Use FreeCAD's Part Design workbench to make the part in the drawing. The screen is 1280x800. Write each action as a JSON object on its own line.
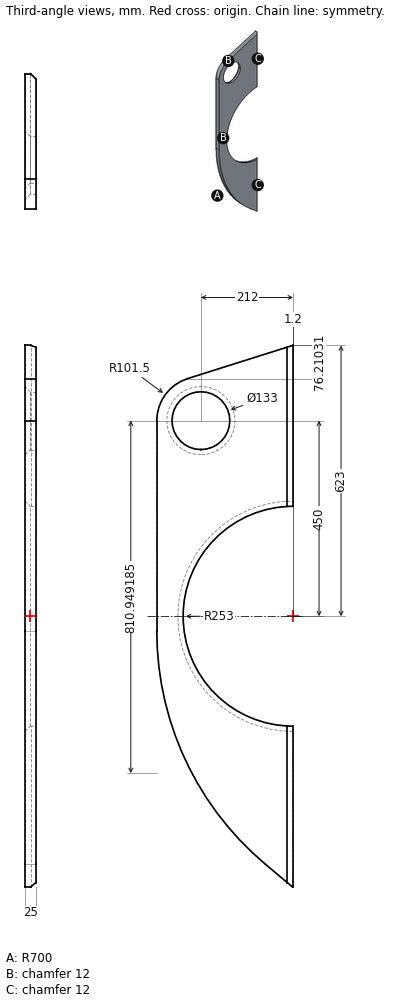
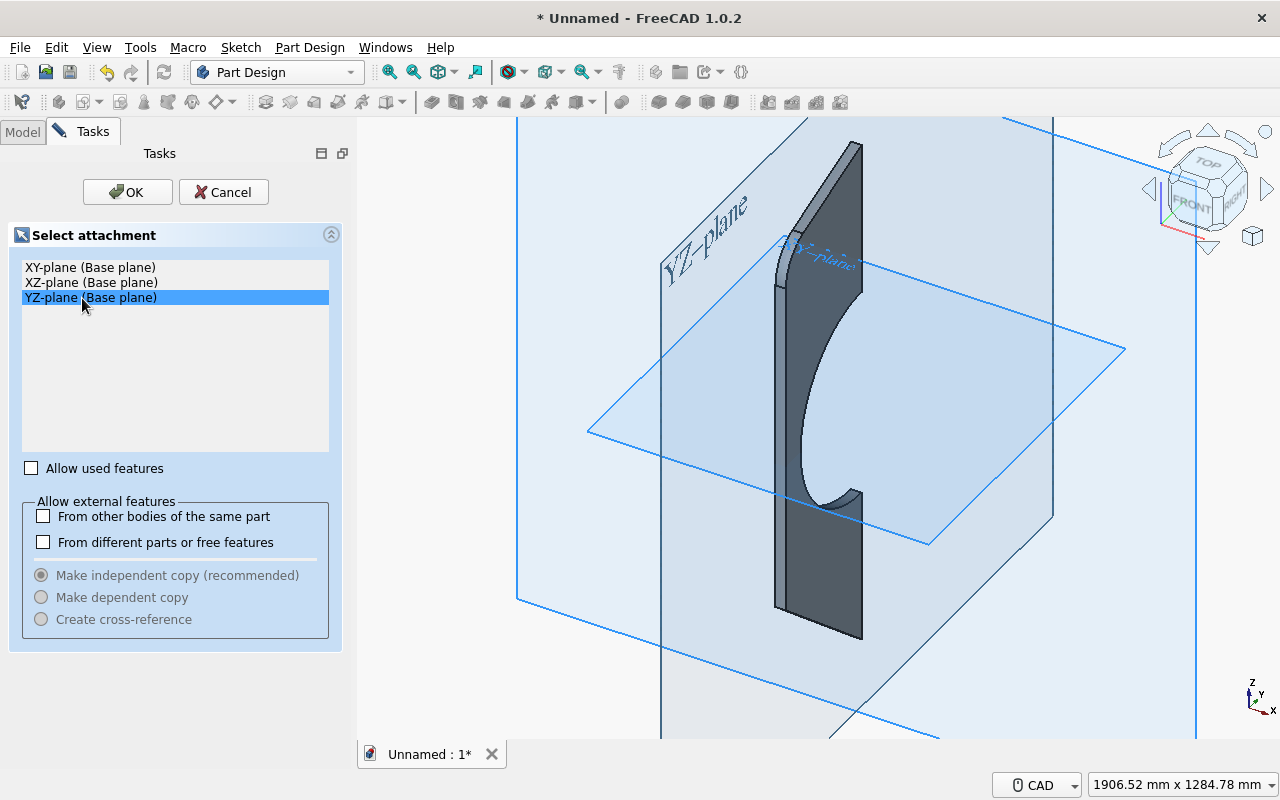
{"action": "left_click", "coordinate": [128, 192]}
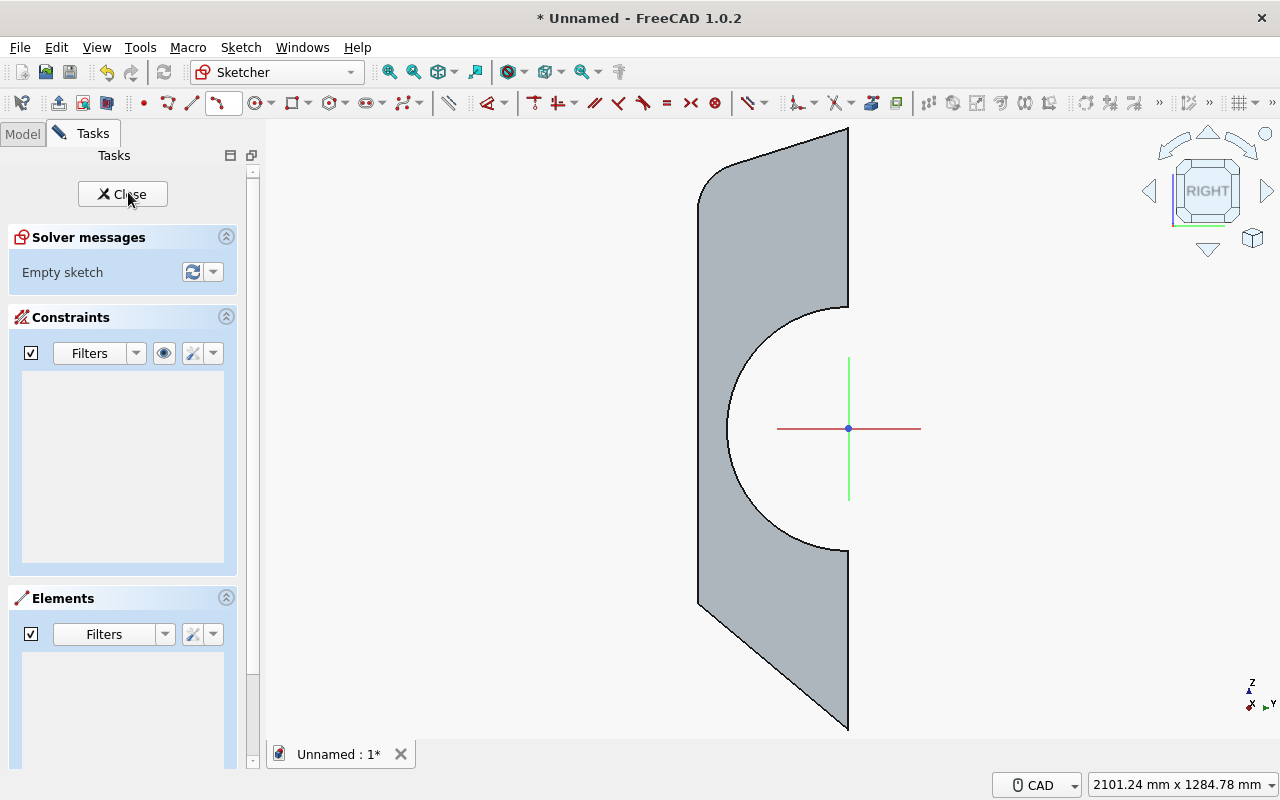
{"action": "left_click", "coordinate": [108, 104]}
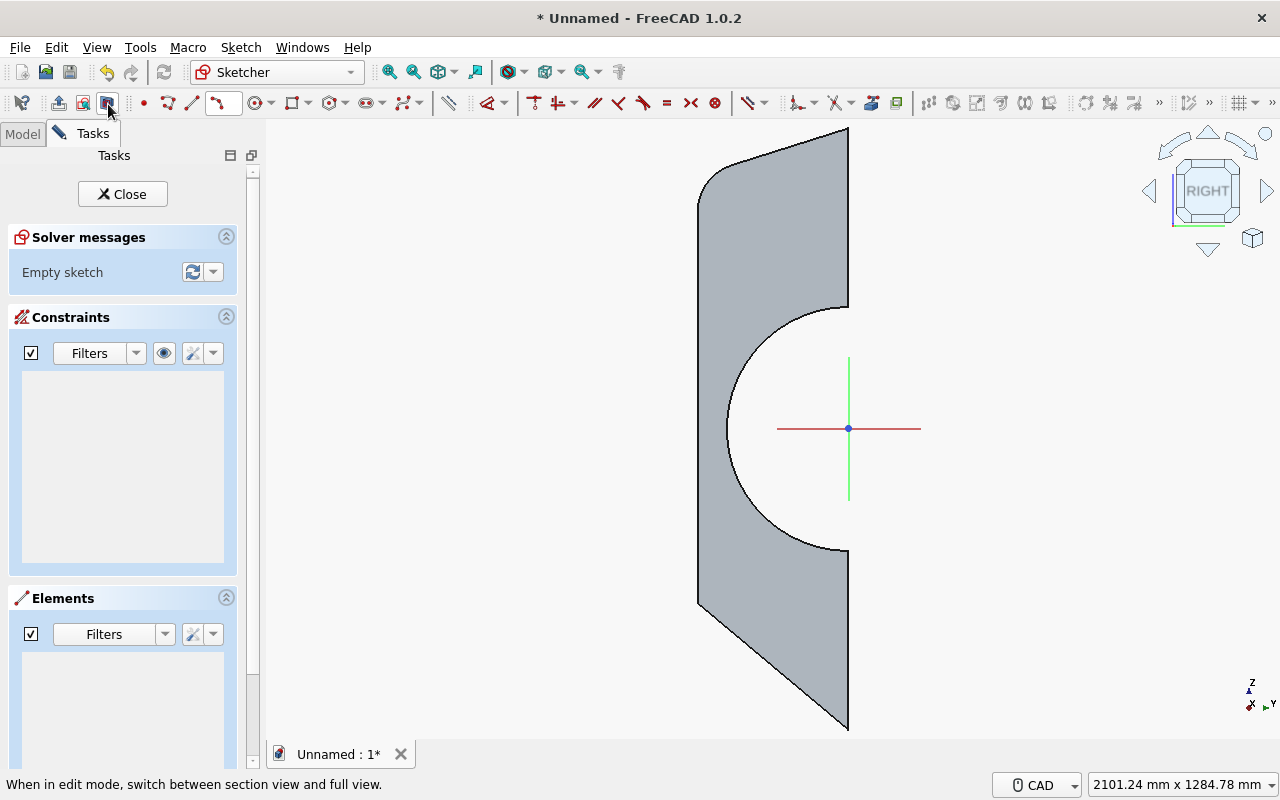
{"action": "scroll", "coordinate": [755, 169], "scroll_direction": "up", "scroll_amount": 9}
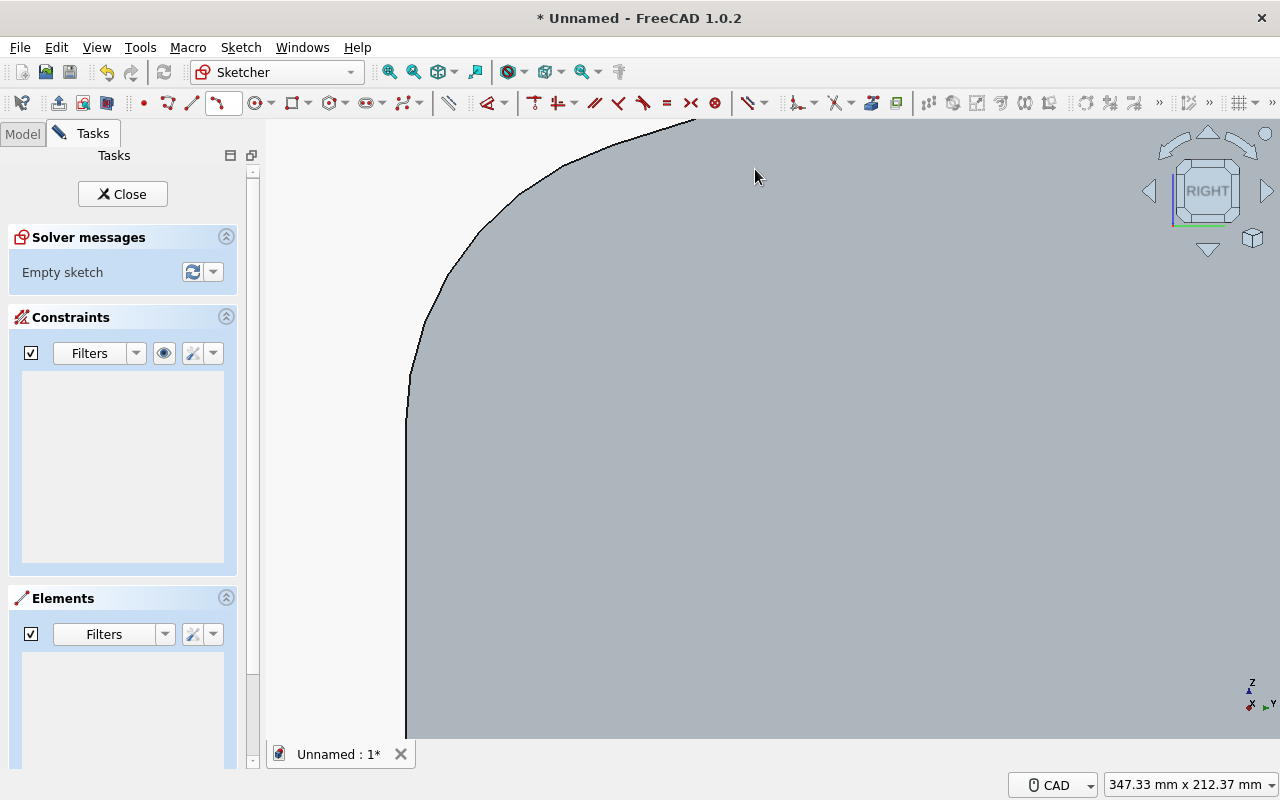
{"action": "left_click", "coordinate": [256, 104]}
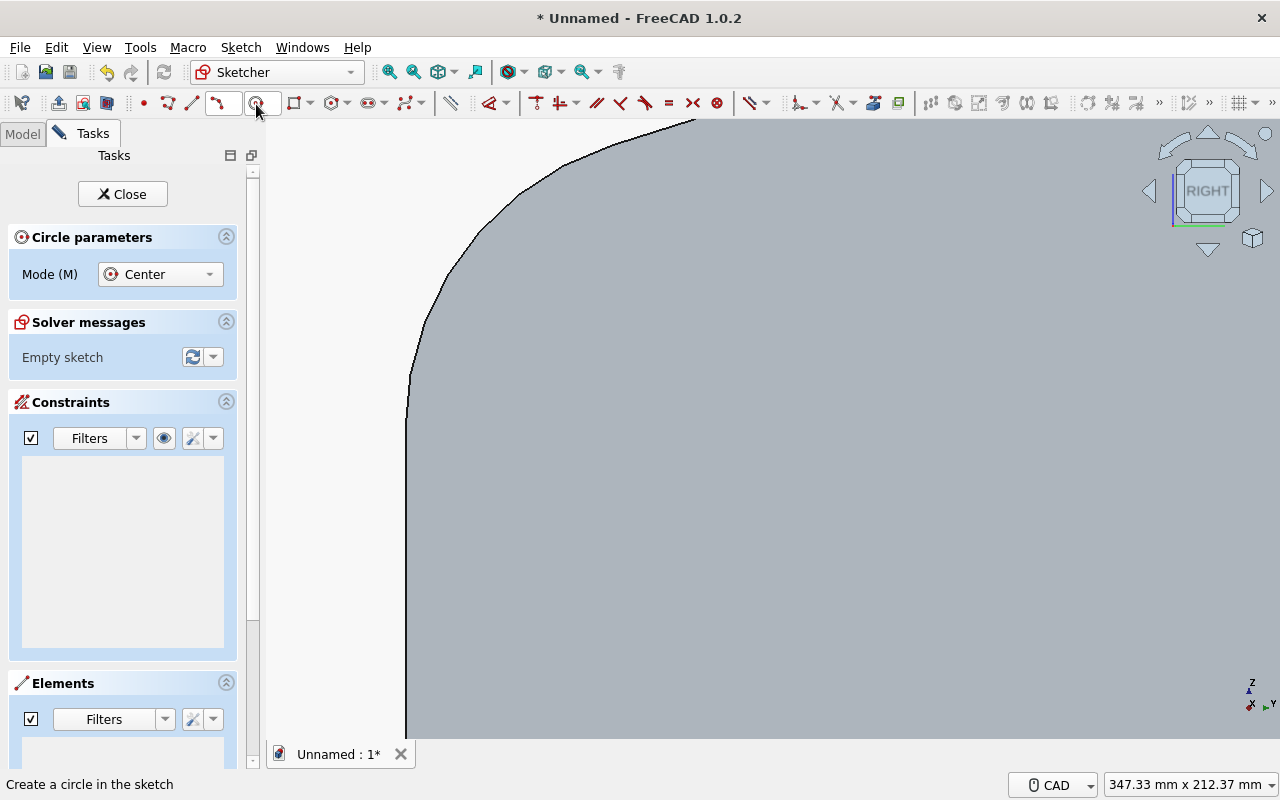
{"action": "left_click", "coordinate": [702, 428]}
{"action": "left_click", "coordinate": [839, 291]}
{"action": "key", "text": "Escape"}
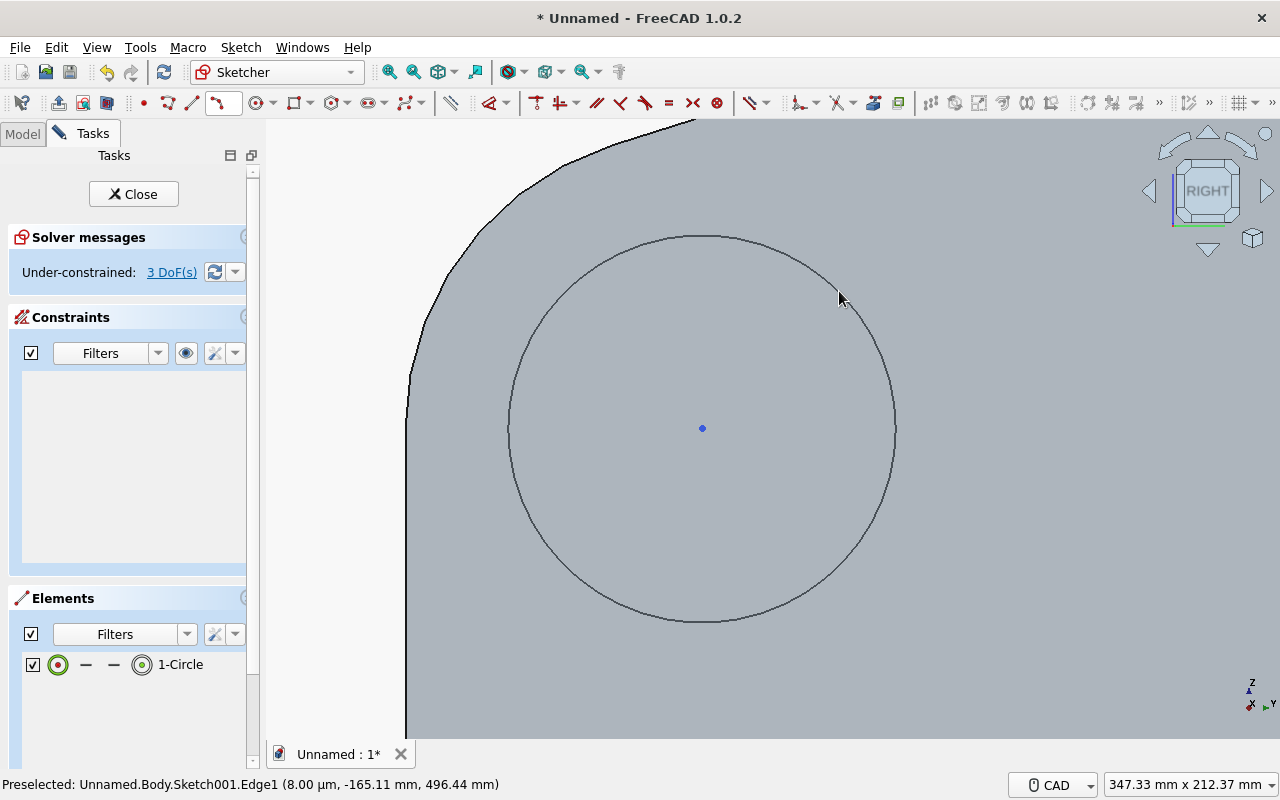
{"action": "left_click", "coordinate": [490, 104]}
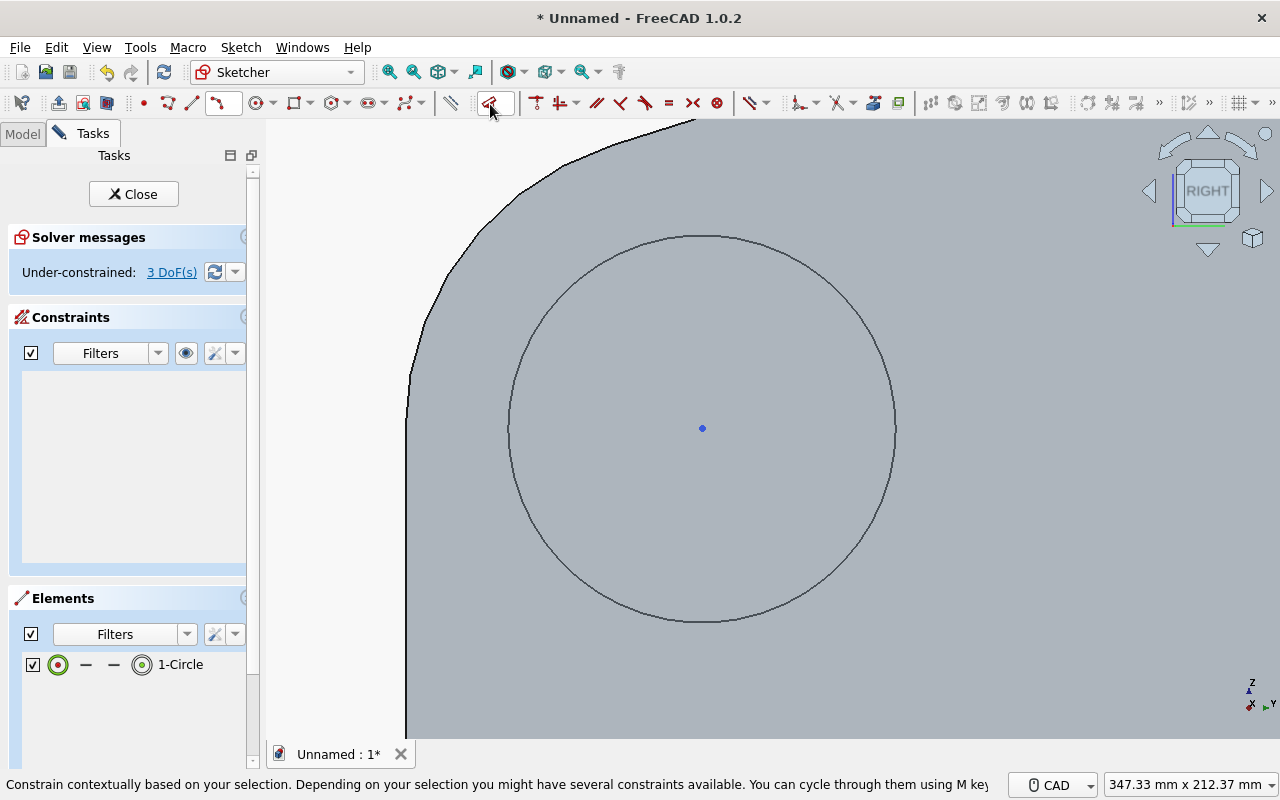
{"action": "left_click", "coordinate": [839, 292]}
{"action": "left_click", "coordinate": [862, 269]}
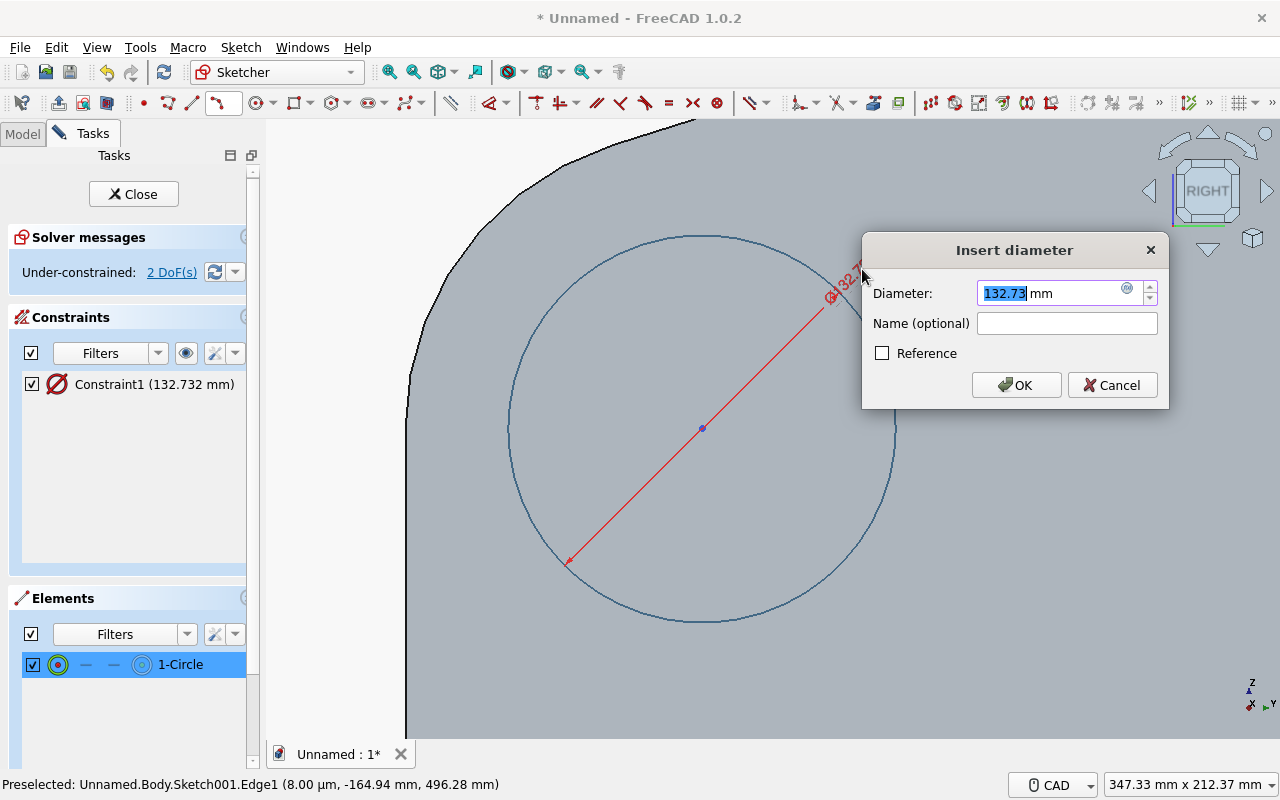
{"action": "type", "text": "133"}
{"action": "key", "text": "Return"}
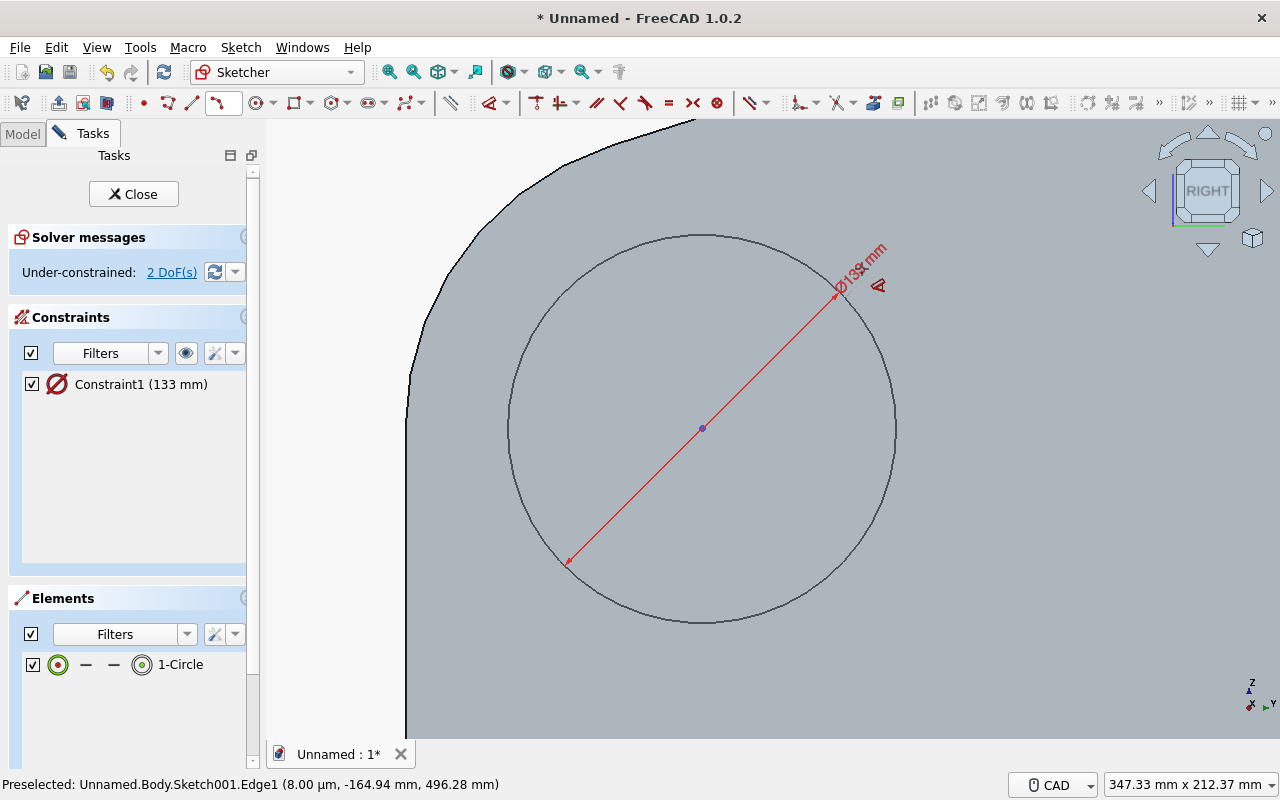
{"action": "left_click", "coordinate": [702, 429]}
{"action": "left_click", "coordinate": [909, 395]}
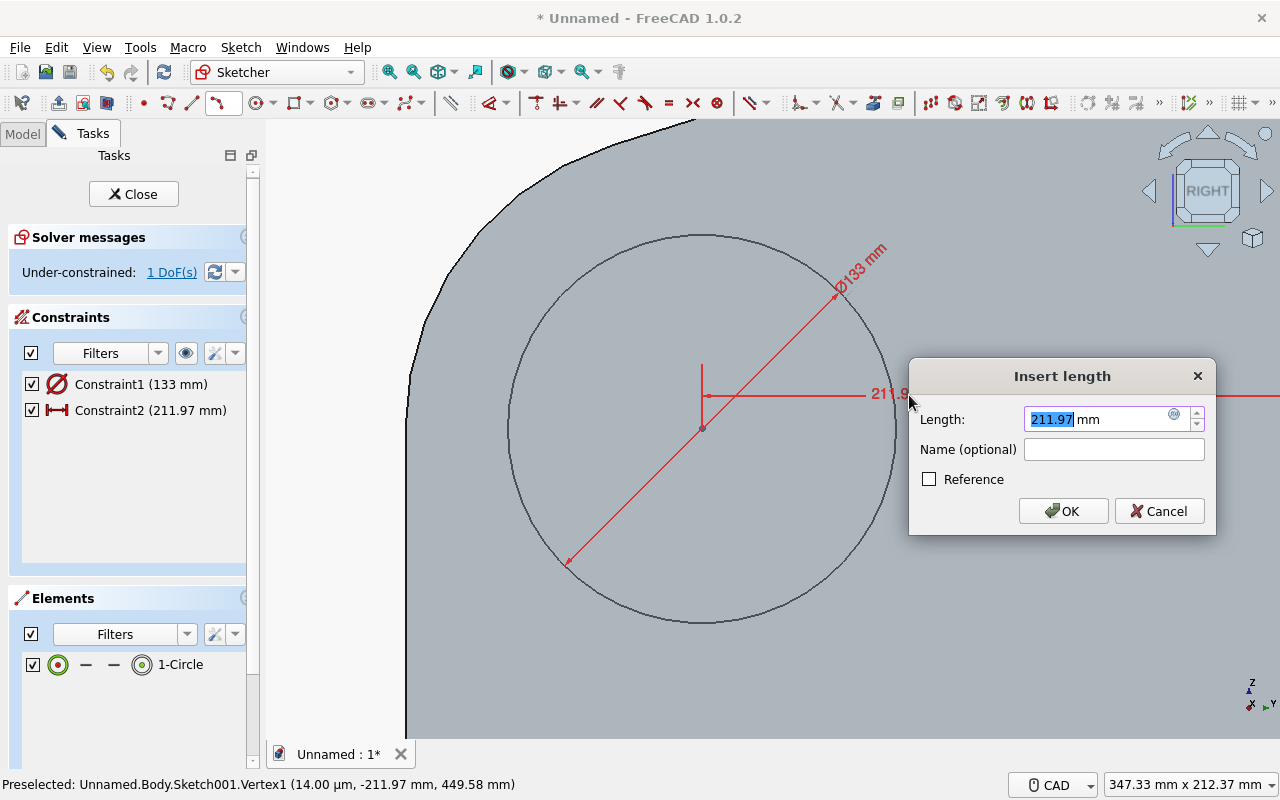
{"action": "type", "text": "212"}
{"action": "key", "text": "Return"}